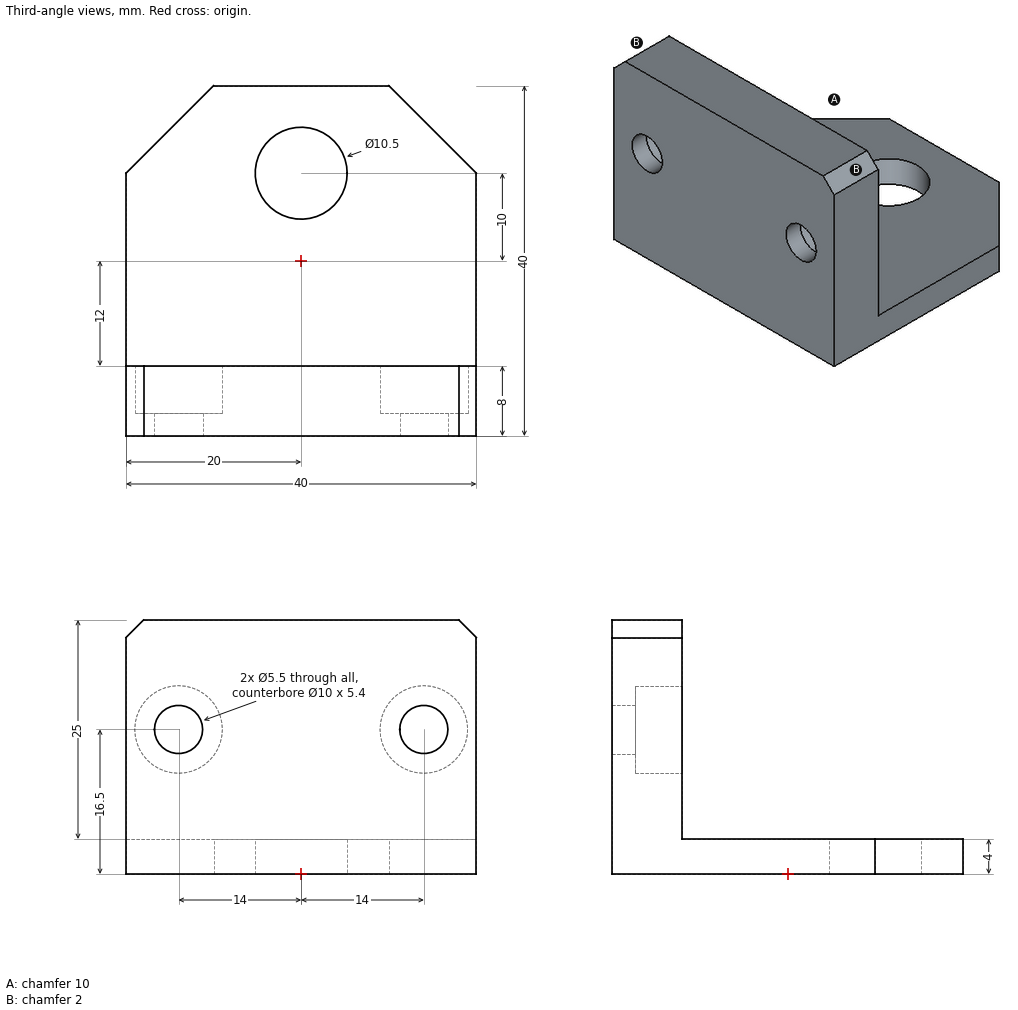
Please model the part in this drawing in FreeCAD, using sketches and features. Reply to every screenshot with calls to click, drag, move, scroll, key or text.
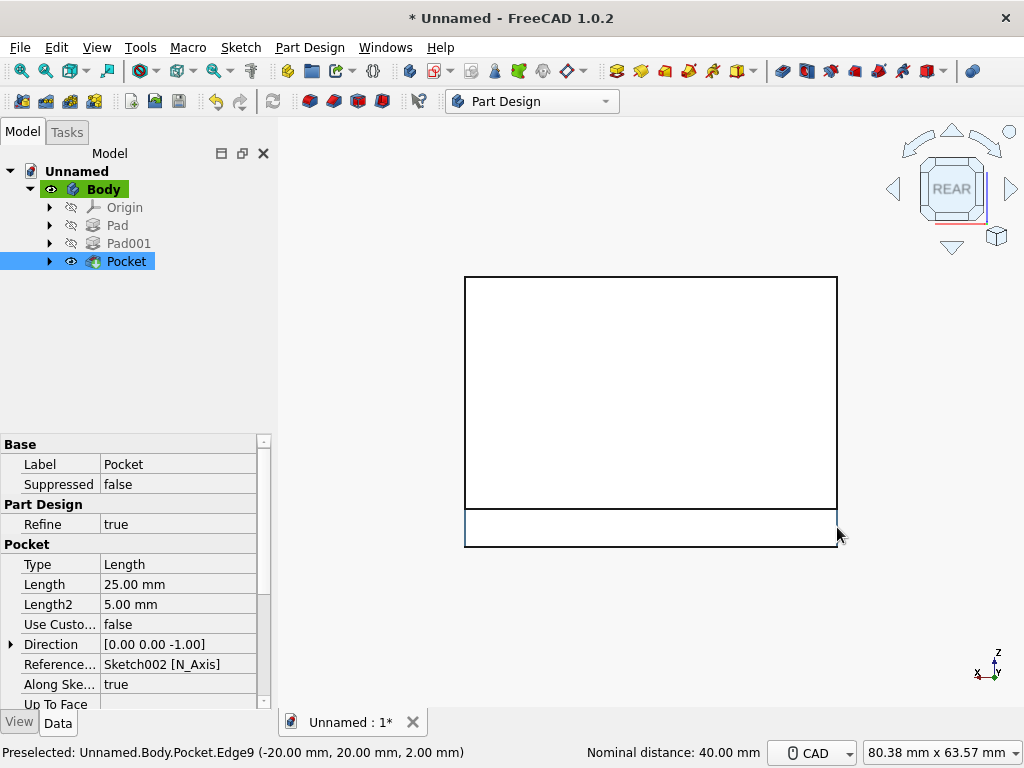
click(334, 102)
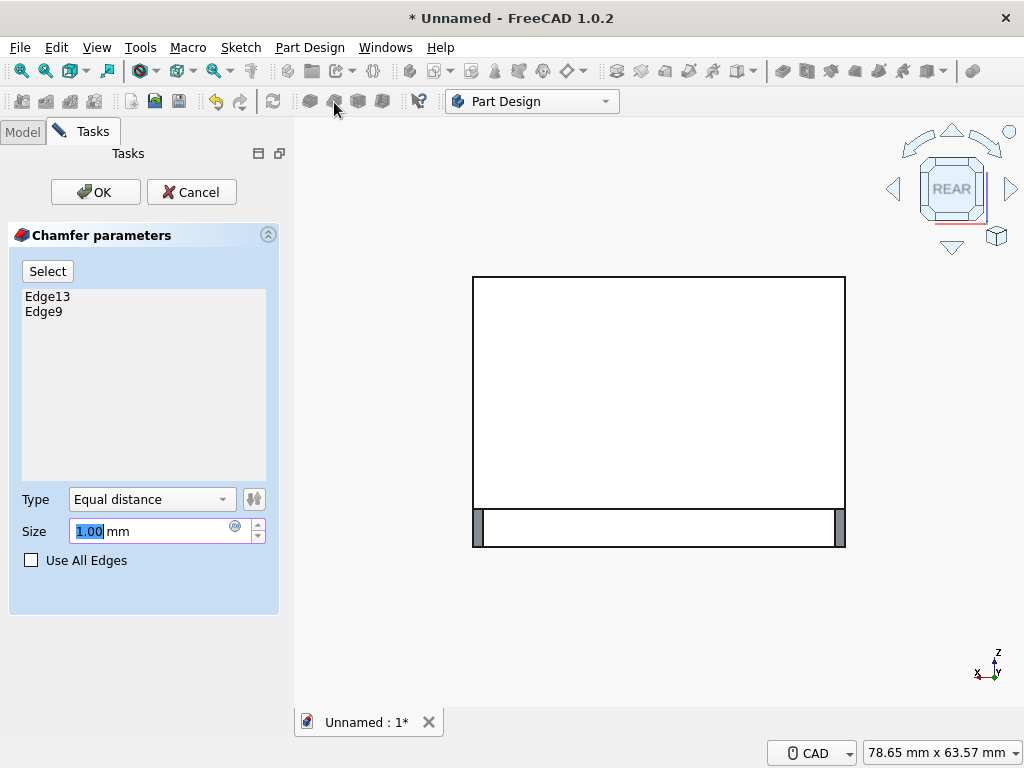
text(10)
key(Tab)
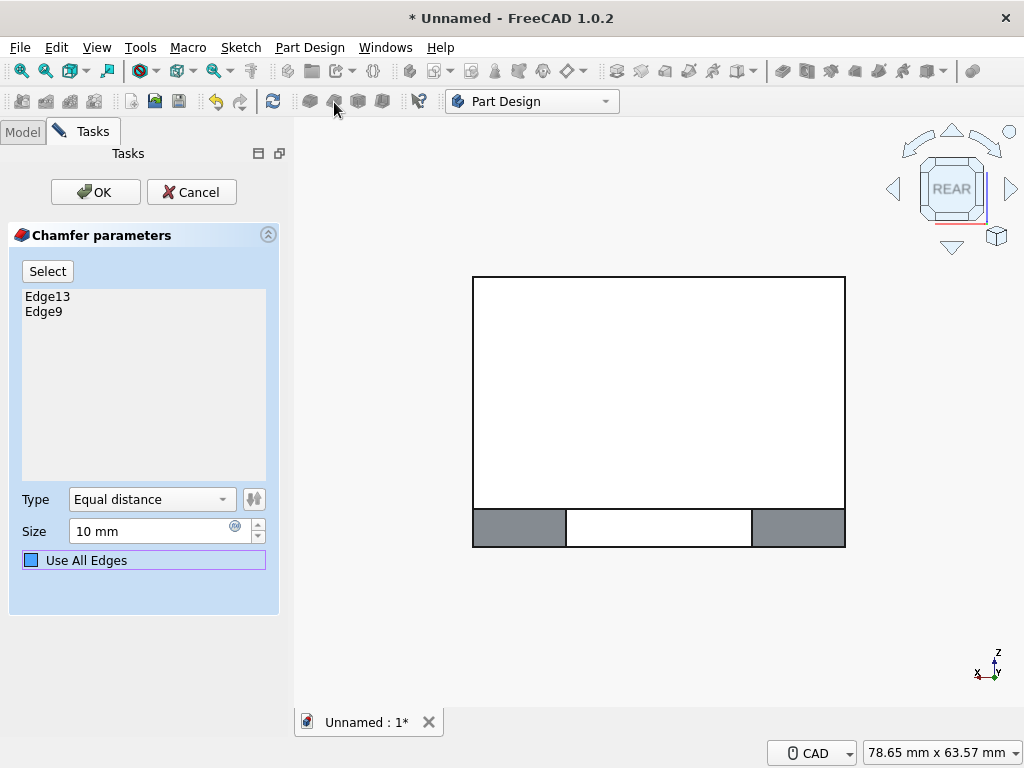
click(96, 192)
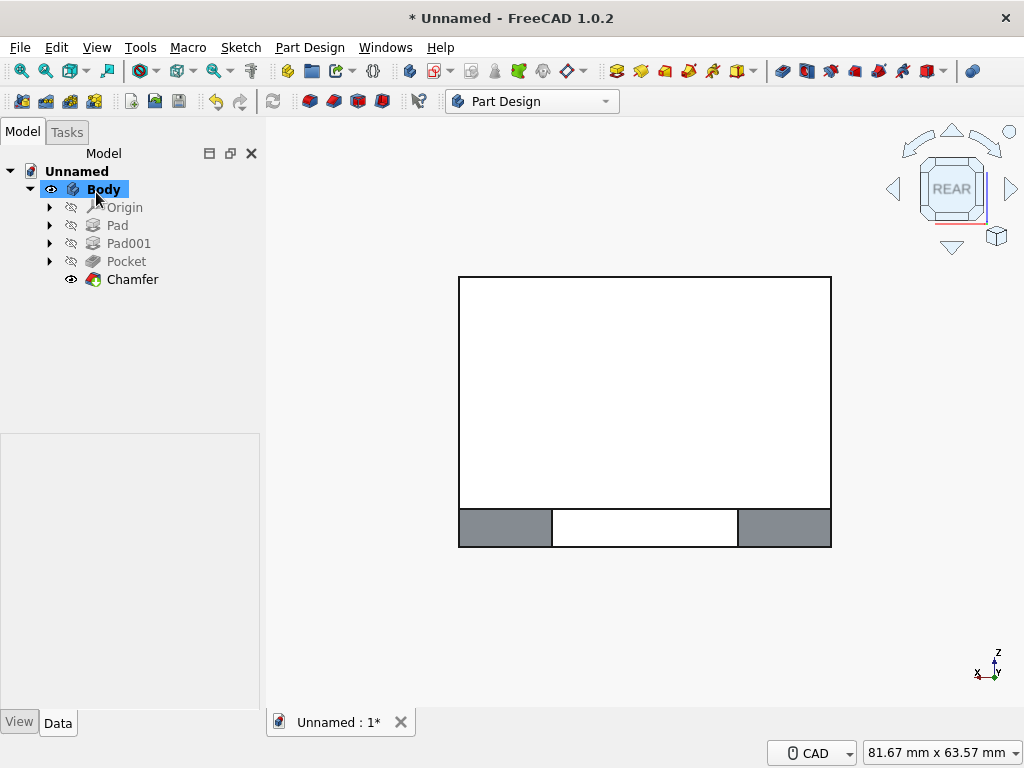
click(592, 392)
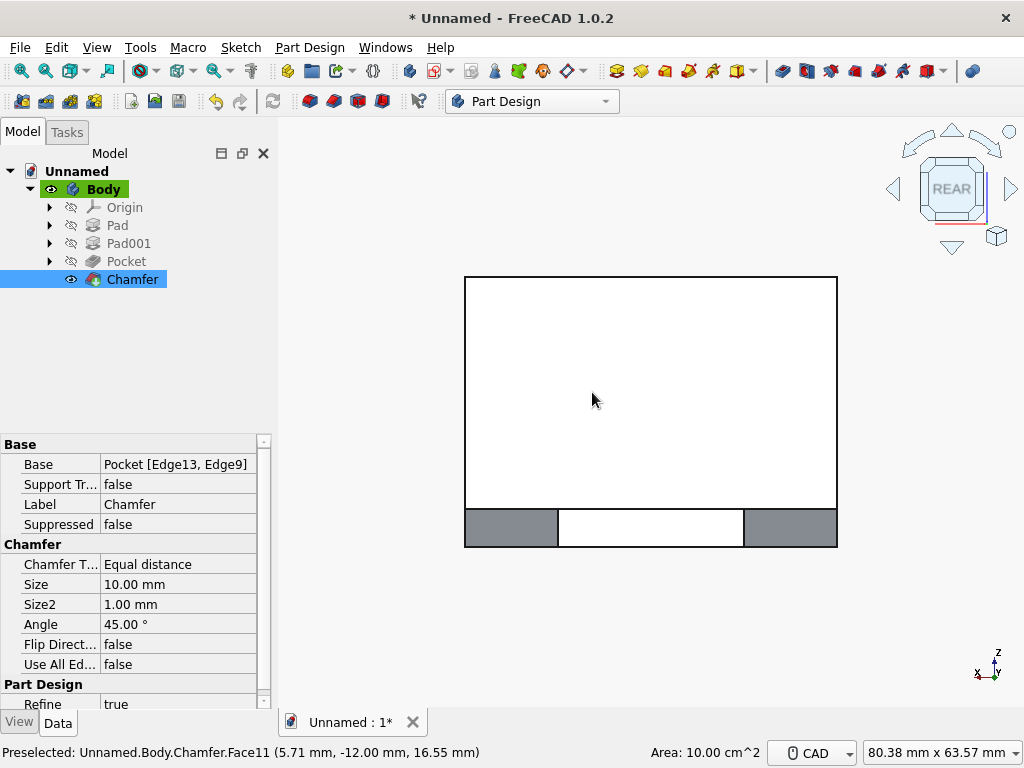
click(434, 72)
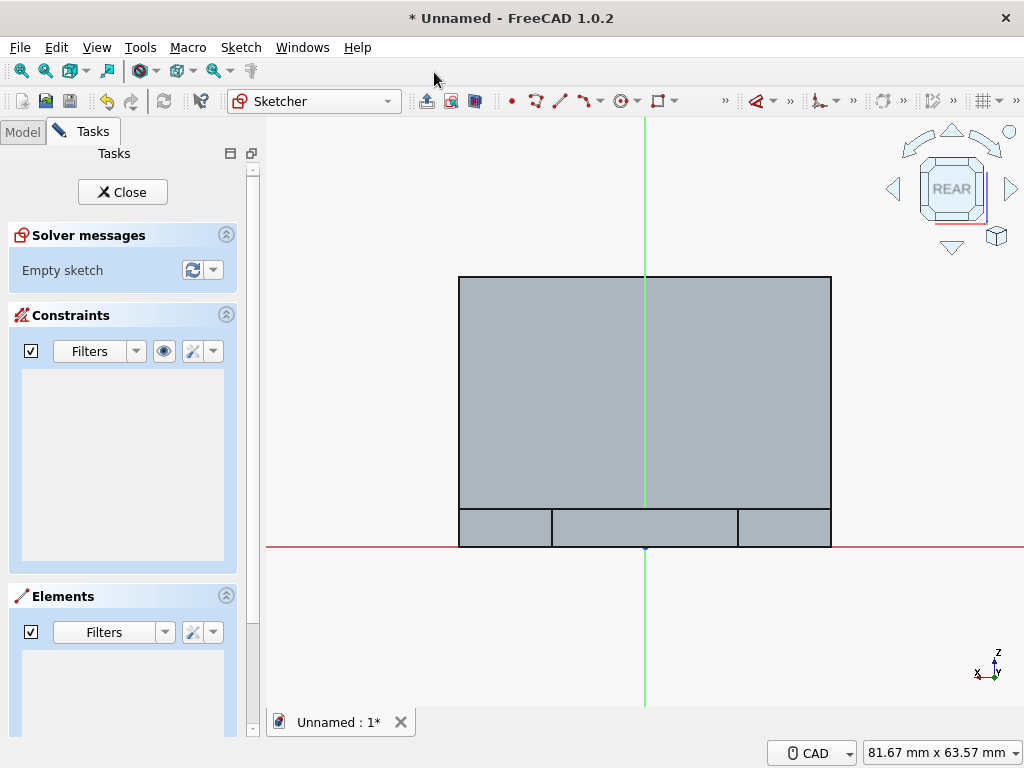
click(476, 102)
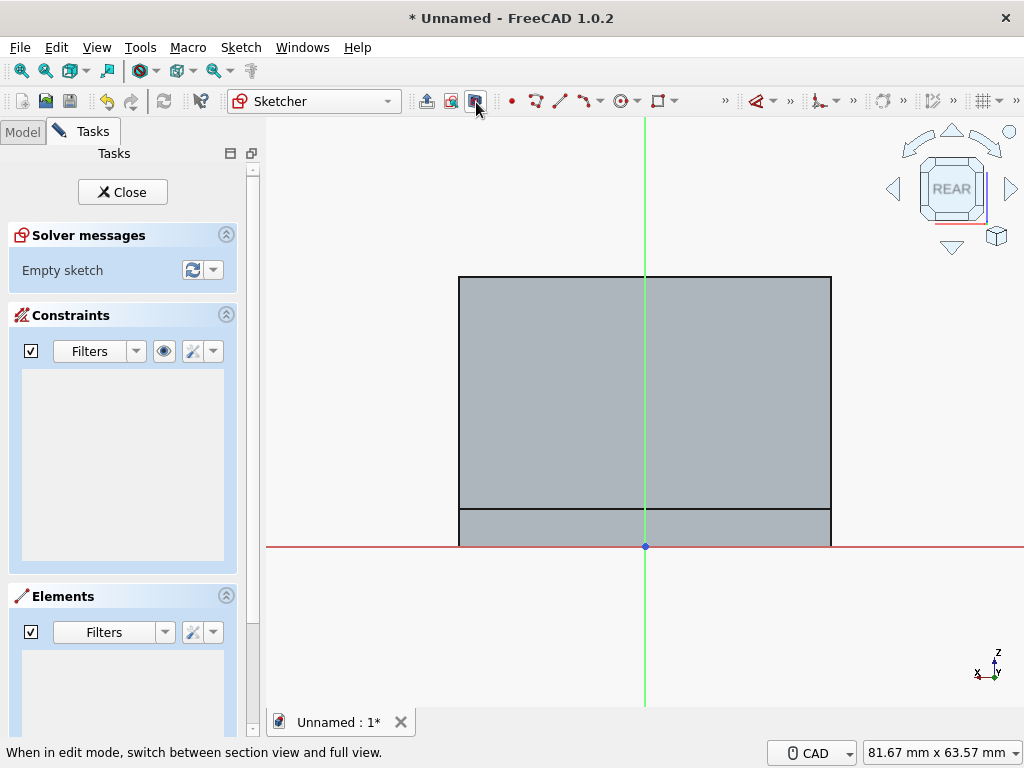
key(g)
key(c)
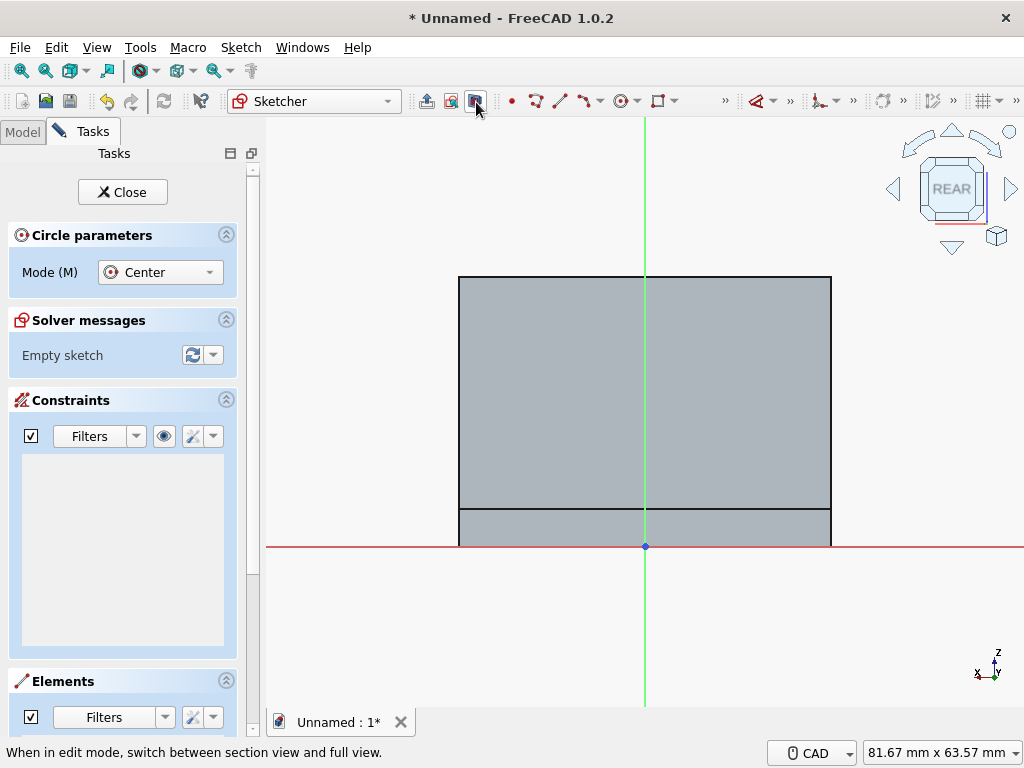
click(775, 393)
move(793, 375)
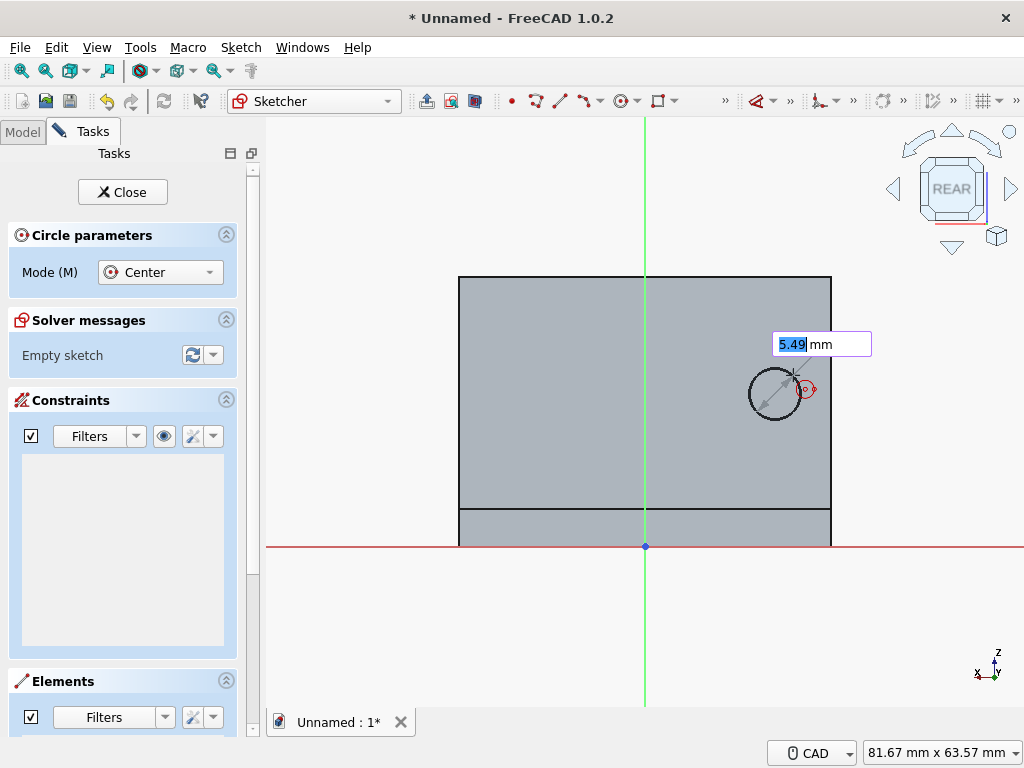
text(5.5)
key(Return)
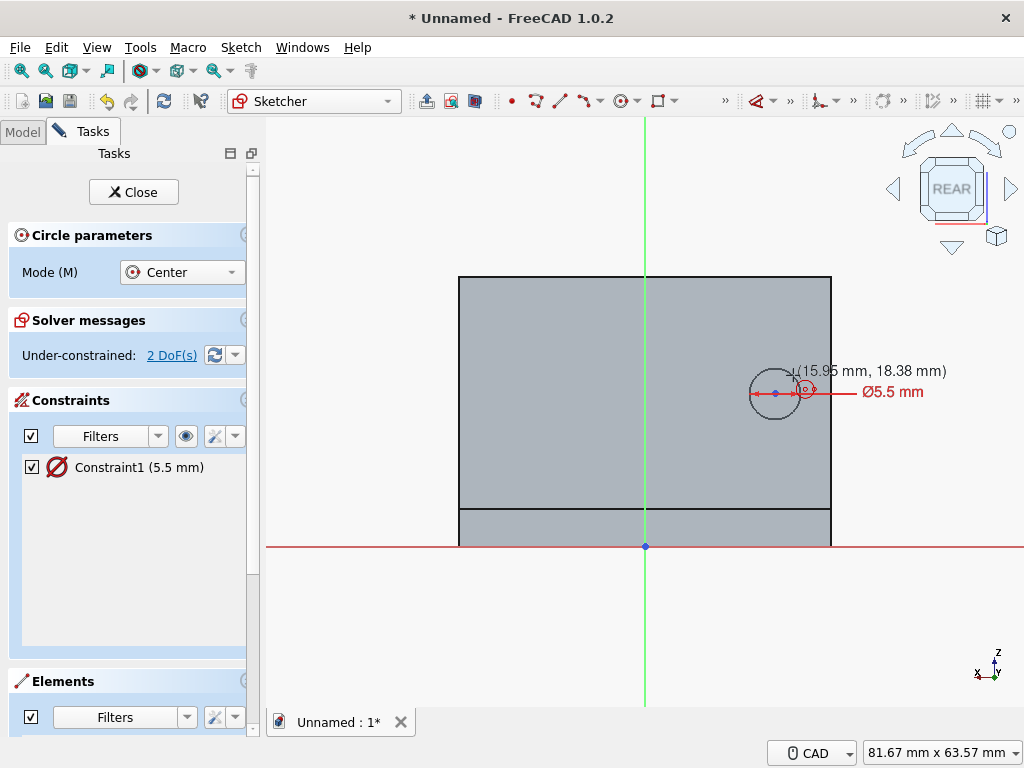
click(515, 393)
move(533, 375)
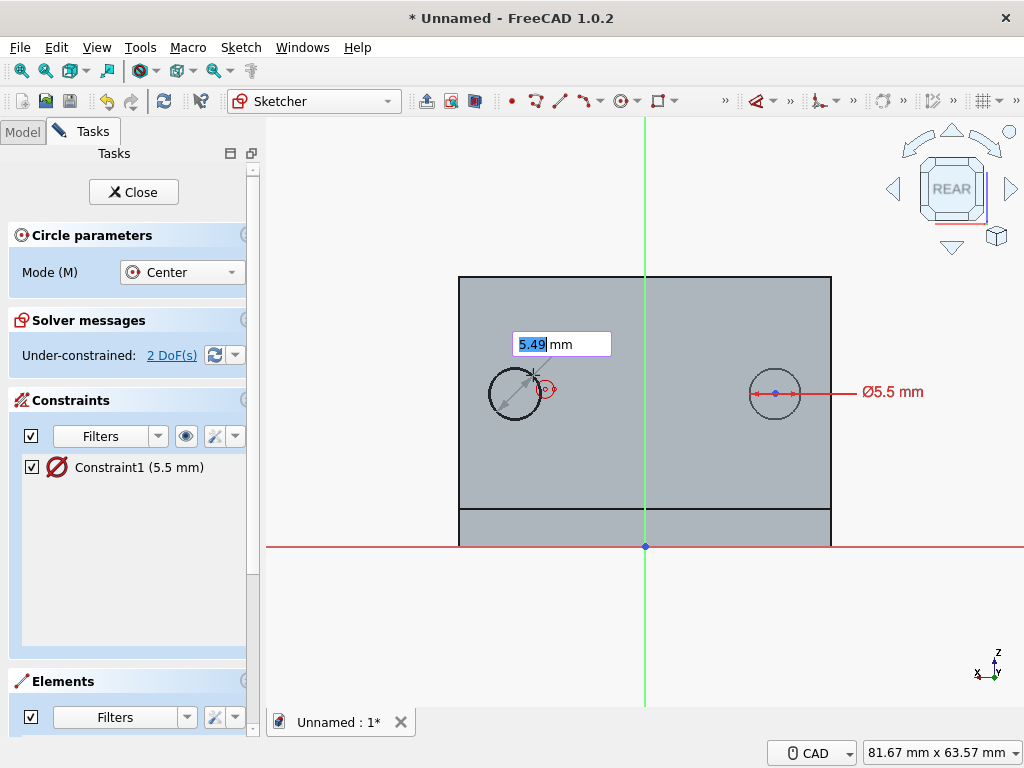
text(5.5)
key(Return)
key(Escape)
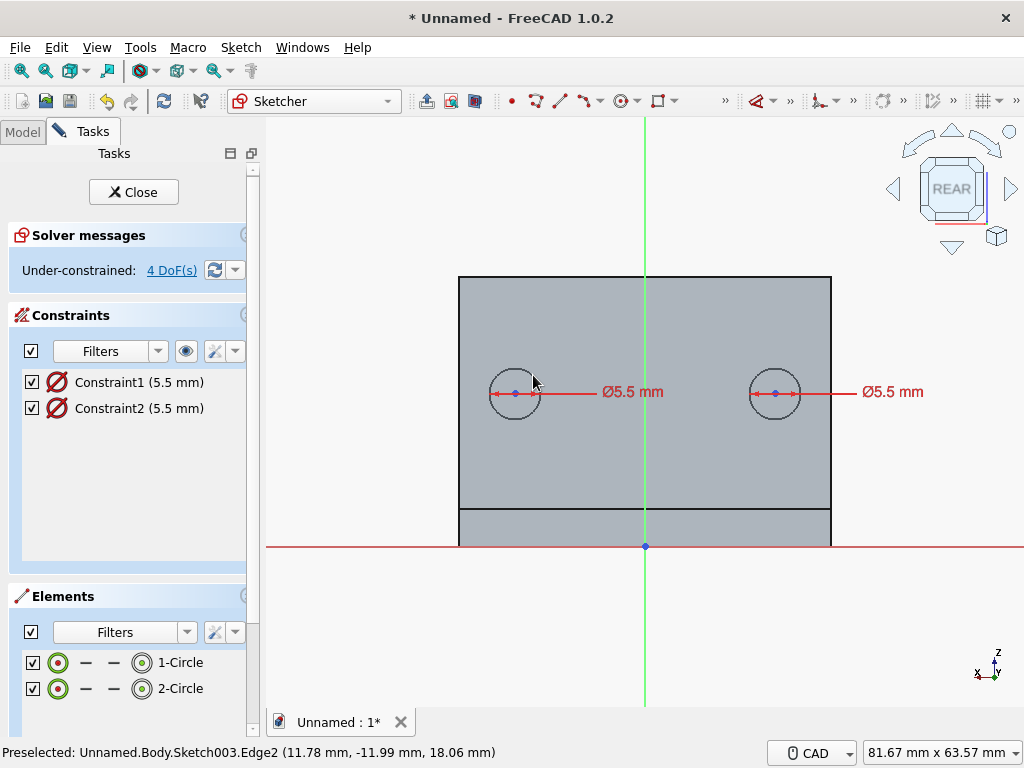
click(756, 102)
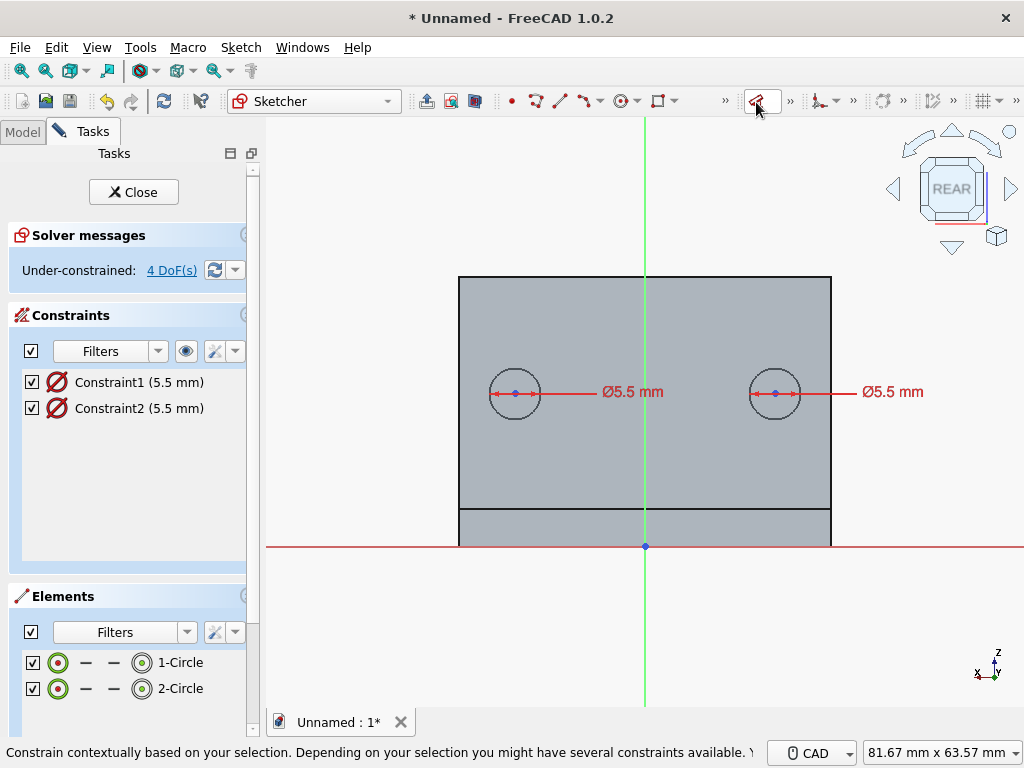
click(775, 394)
click(710, 581)